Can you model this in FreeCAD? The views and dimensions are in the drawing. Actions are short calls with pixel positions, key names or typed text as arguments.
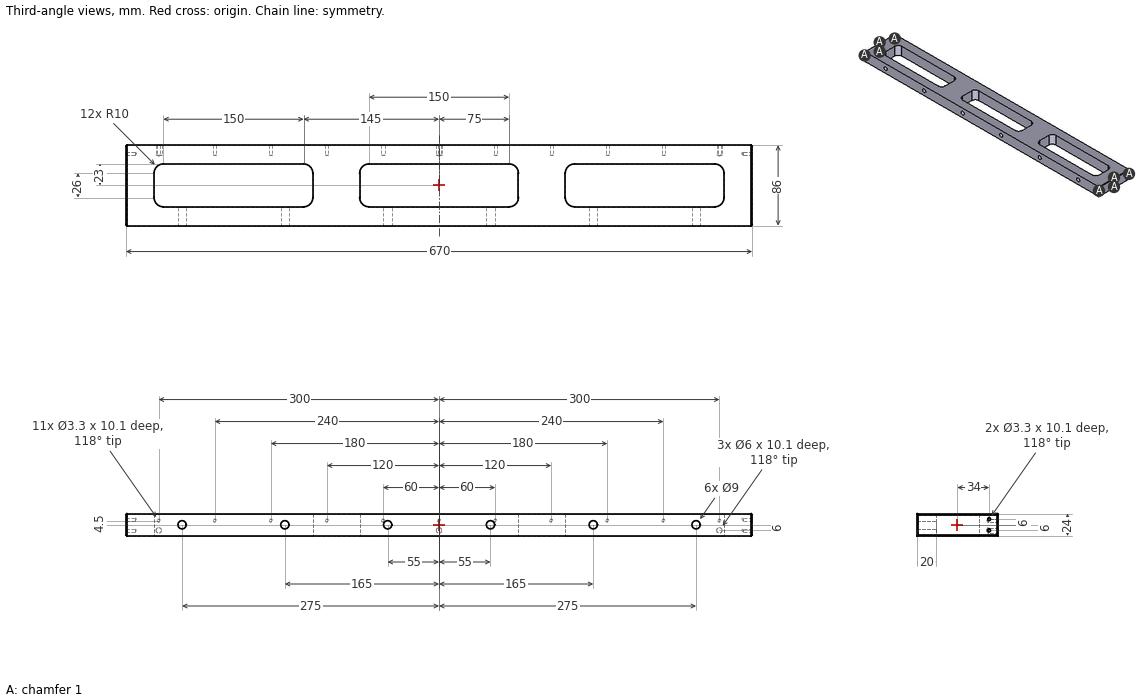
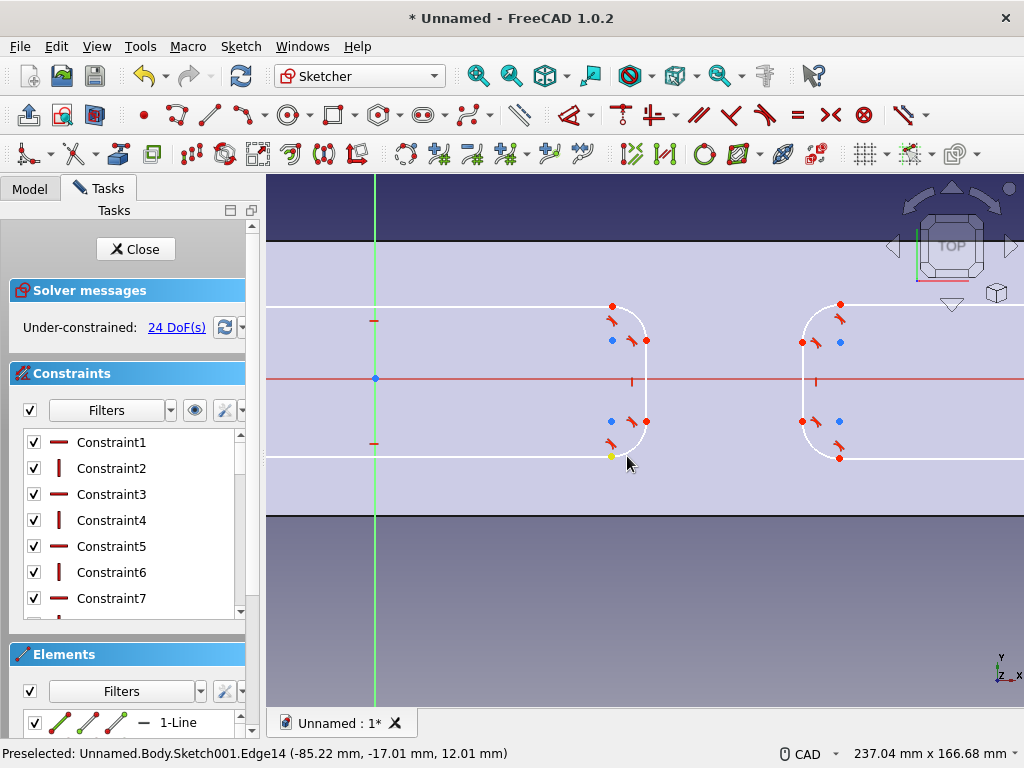
click(627, 453)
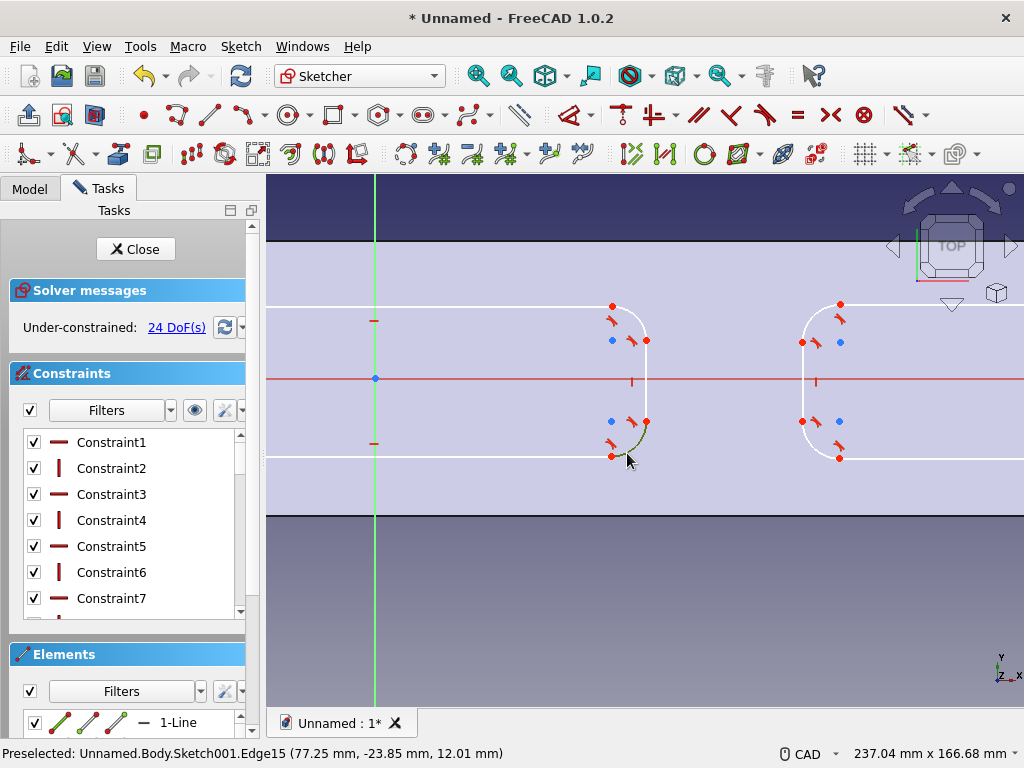
click(643, 325)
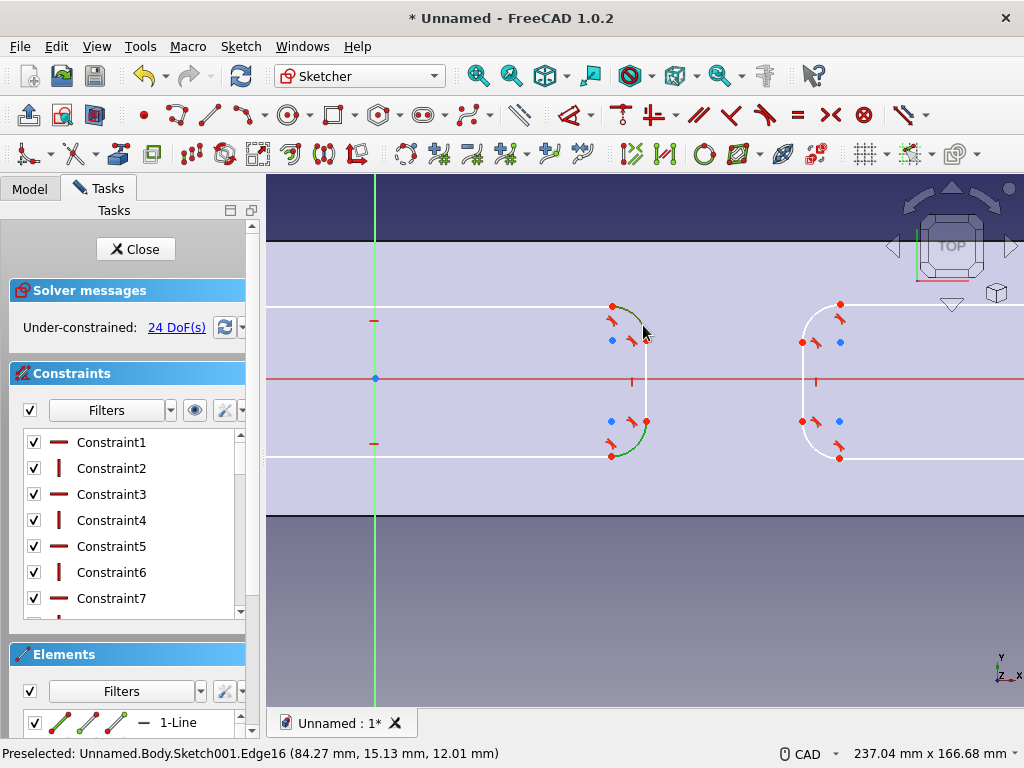
click(823, 309)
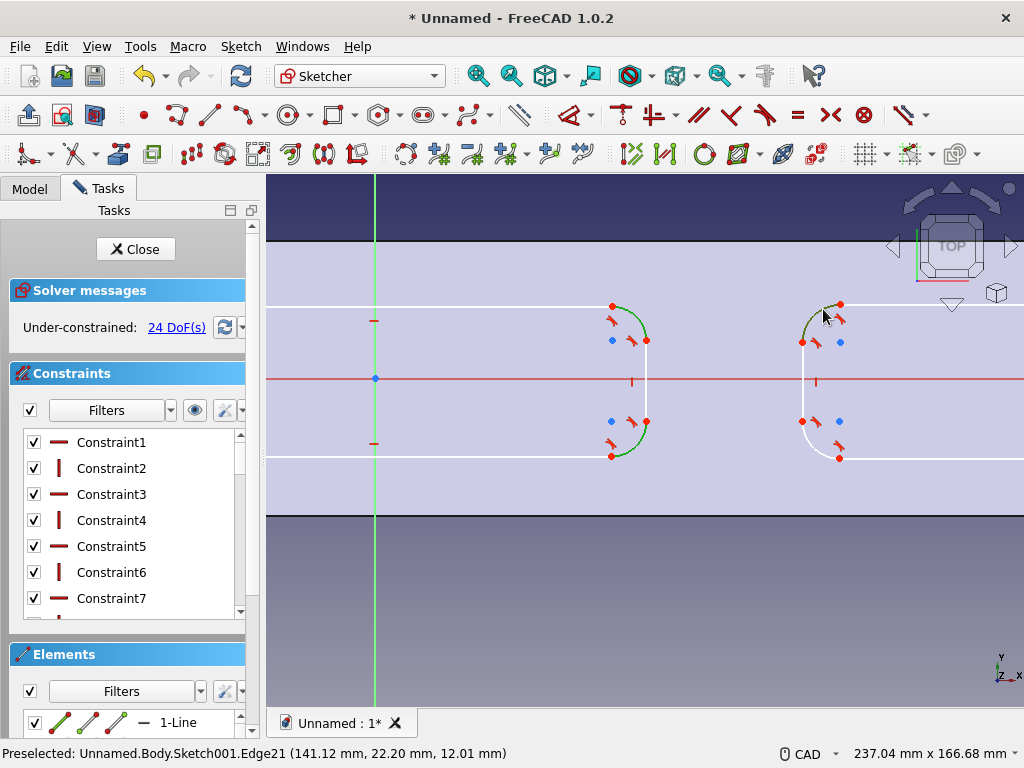
click(807, 439)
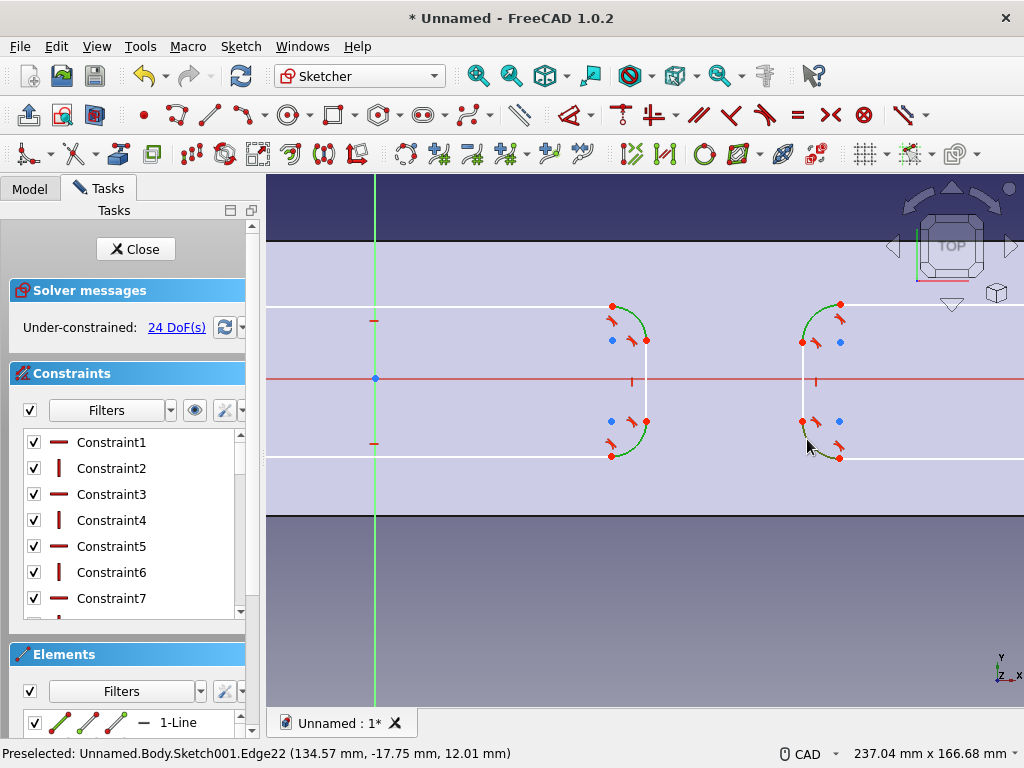
scroll(627, 456, down, 8)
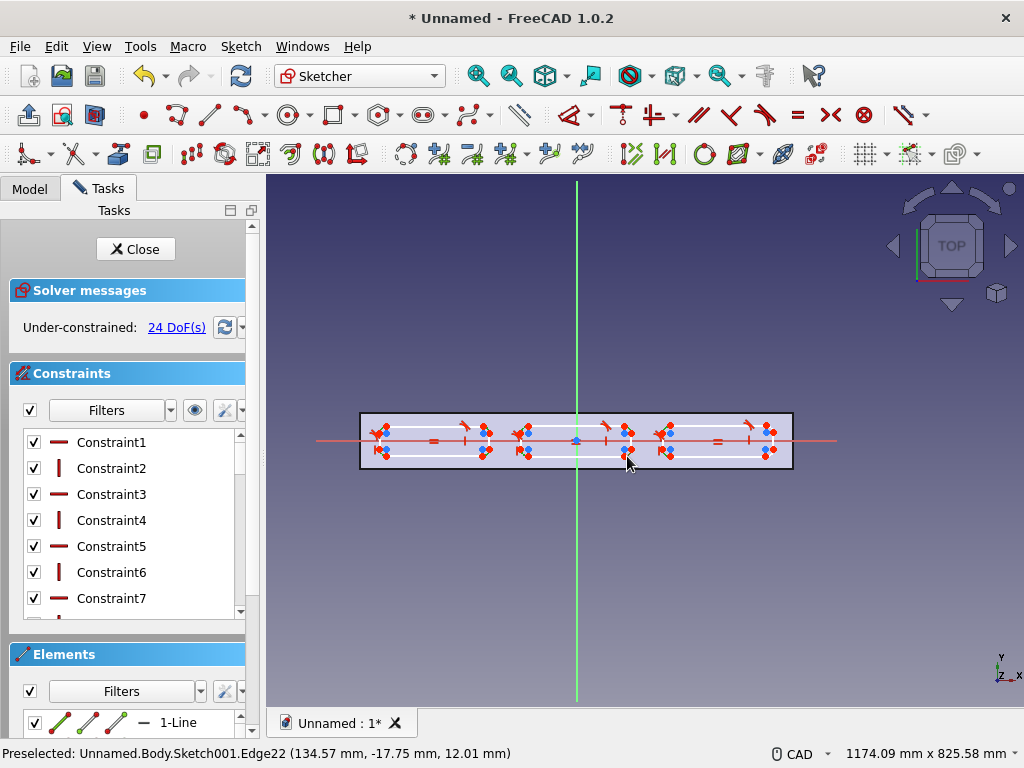
scroll(769, 456, up, 7)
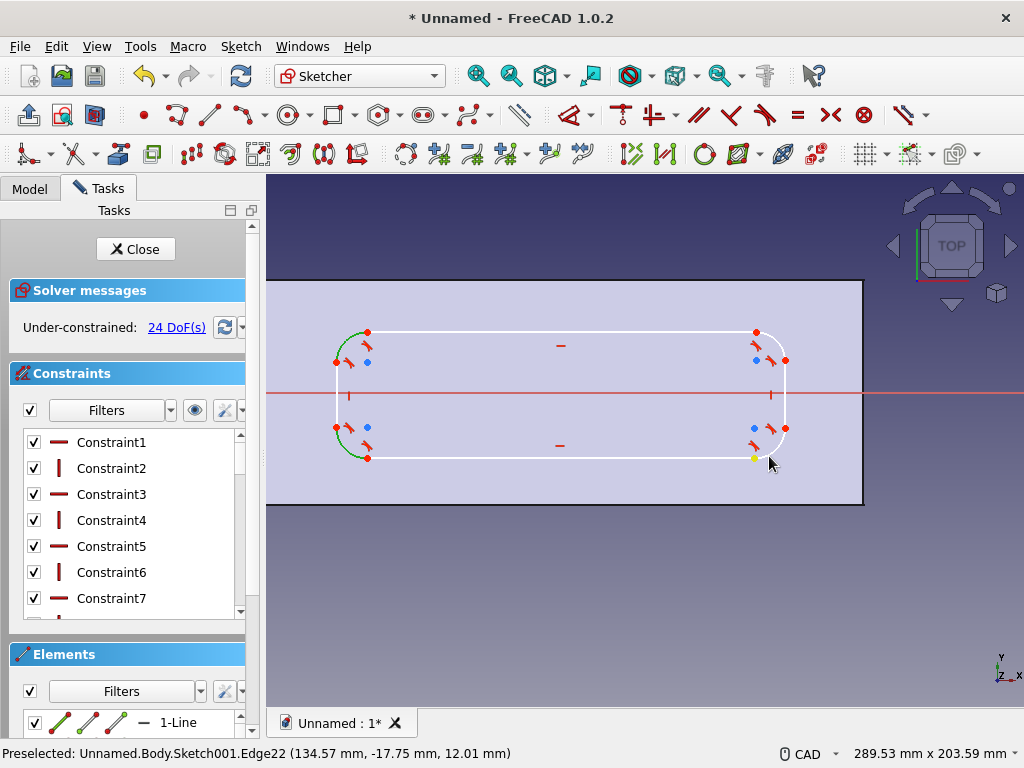
click(768, 455)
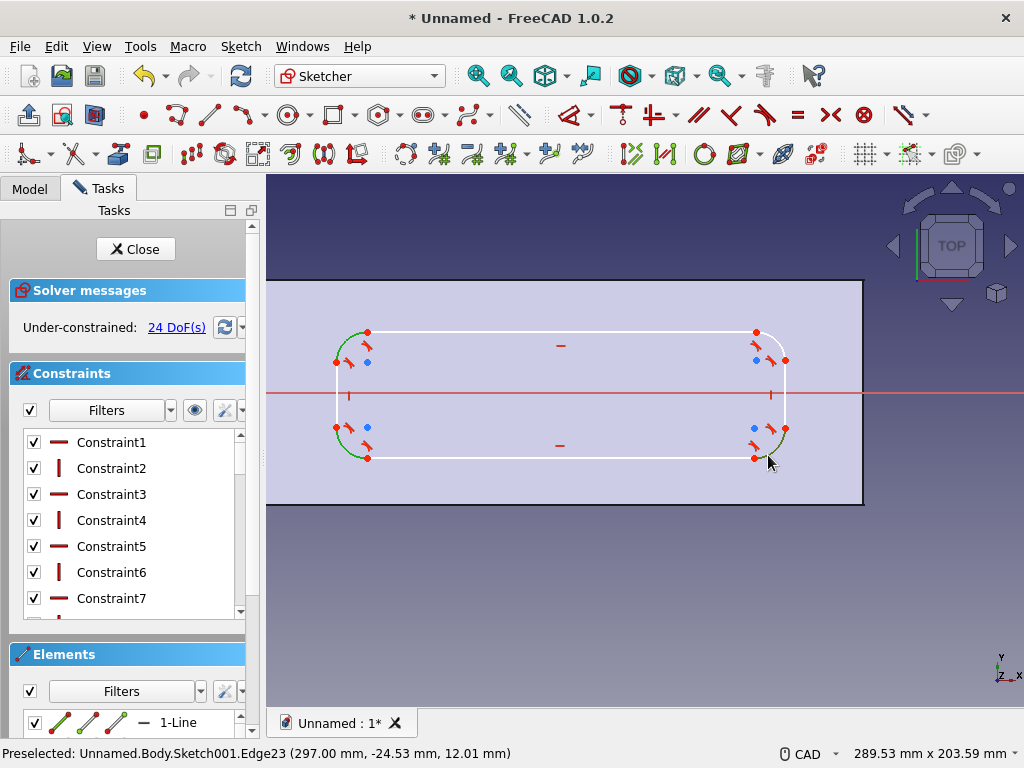
click(782, 348)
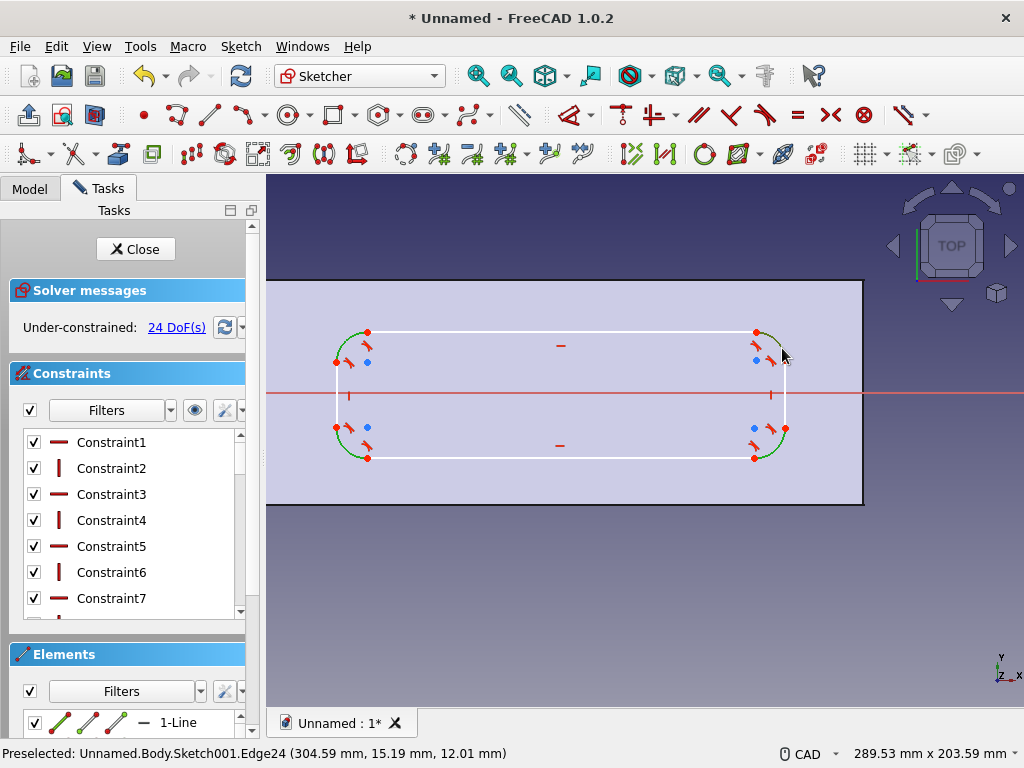
key(e)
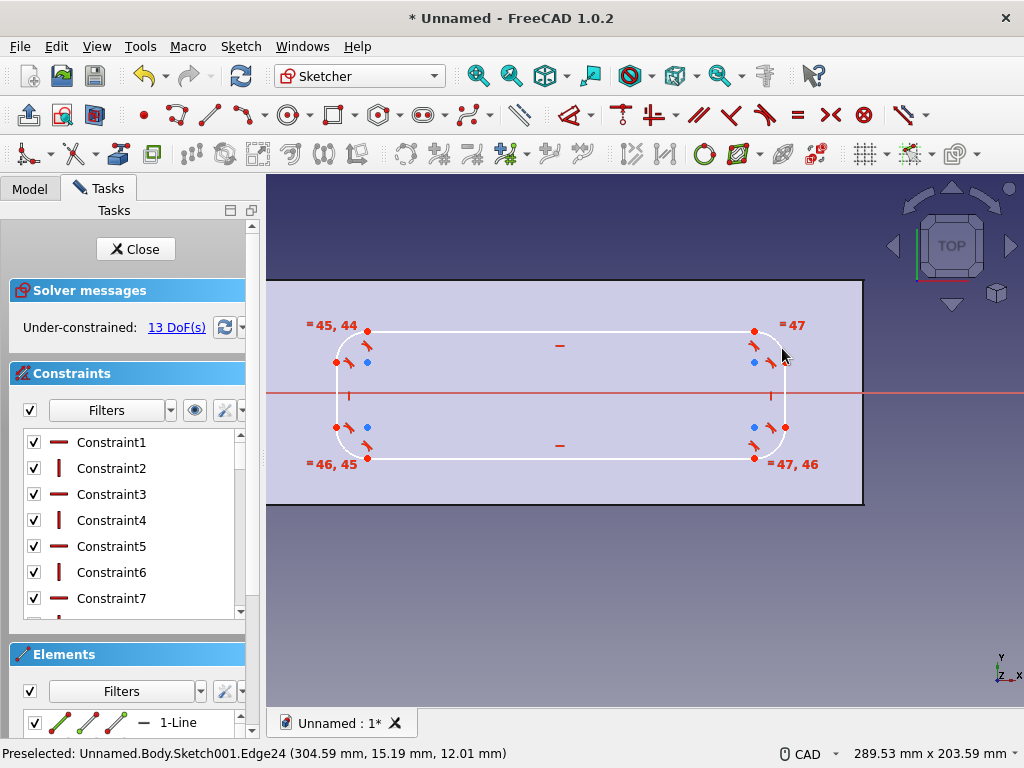
scroll(770, 456, down, 7)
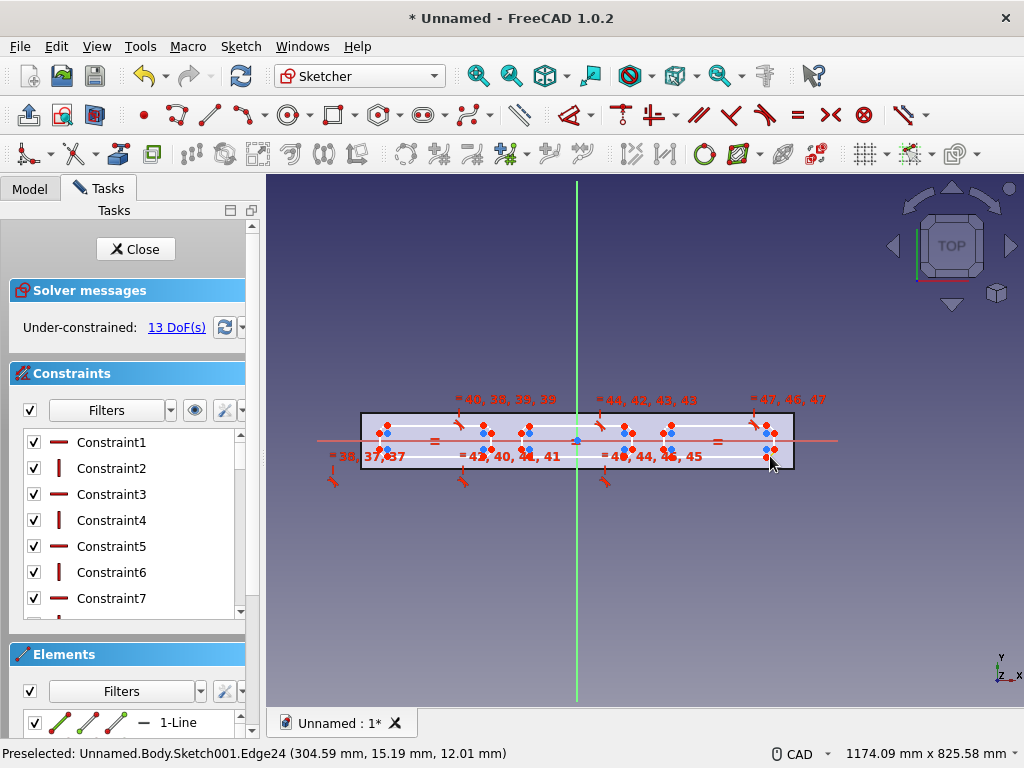
scroll(484, 433, up, 3)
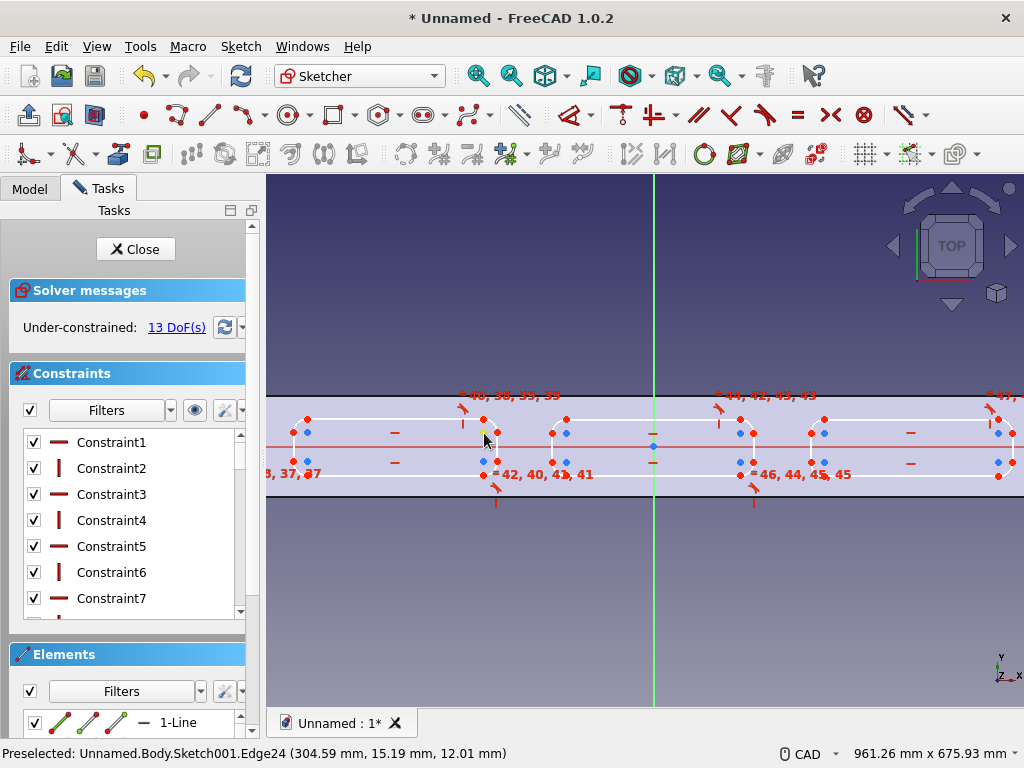
click(483, 433)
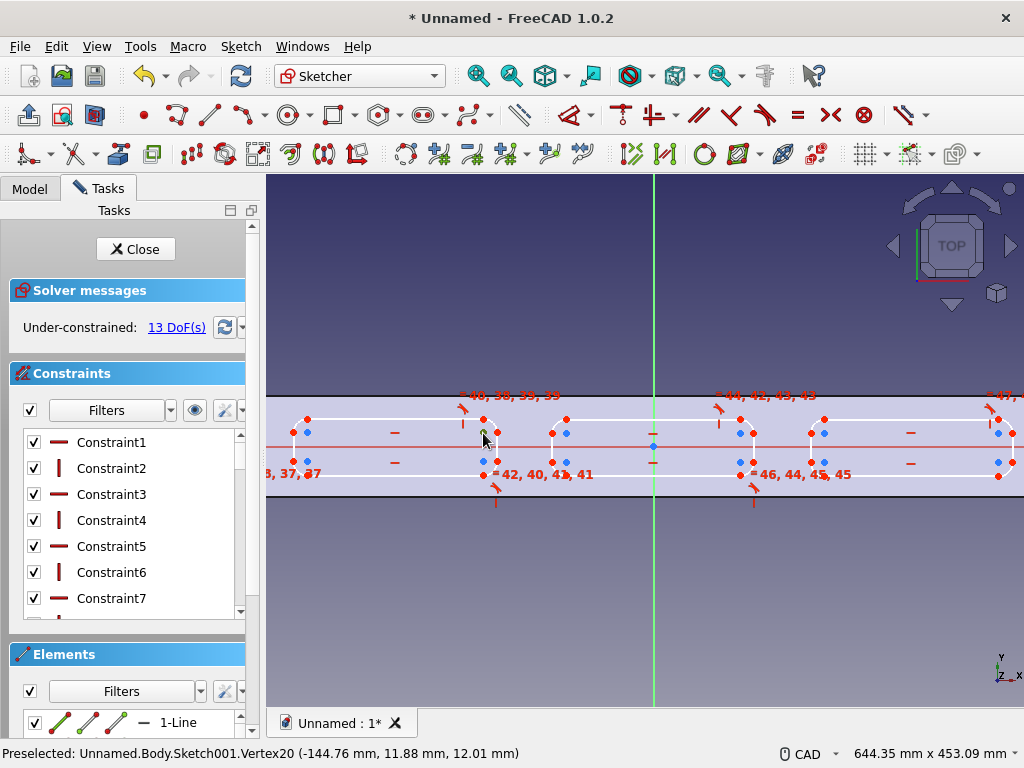
click(825, 433)